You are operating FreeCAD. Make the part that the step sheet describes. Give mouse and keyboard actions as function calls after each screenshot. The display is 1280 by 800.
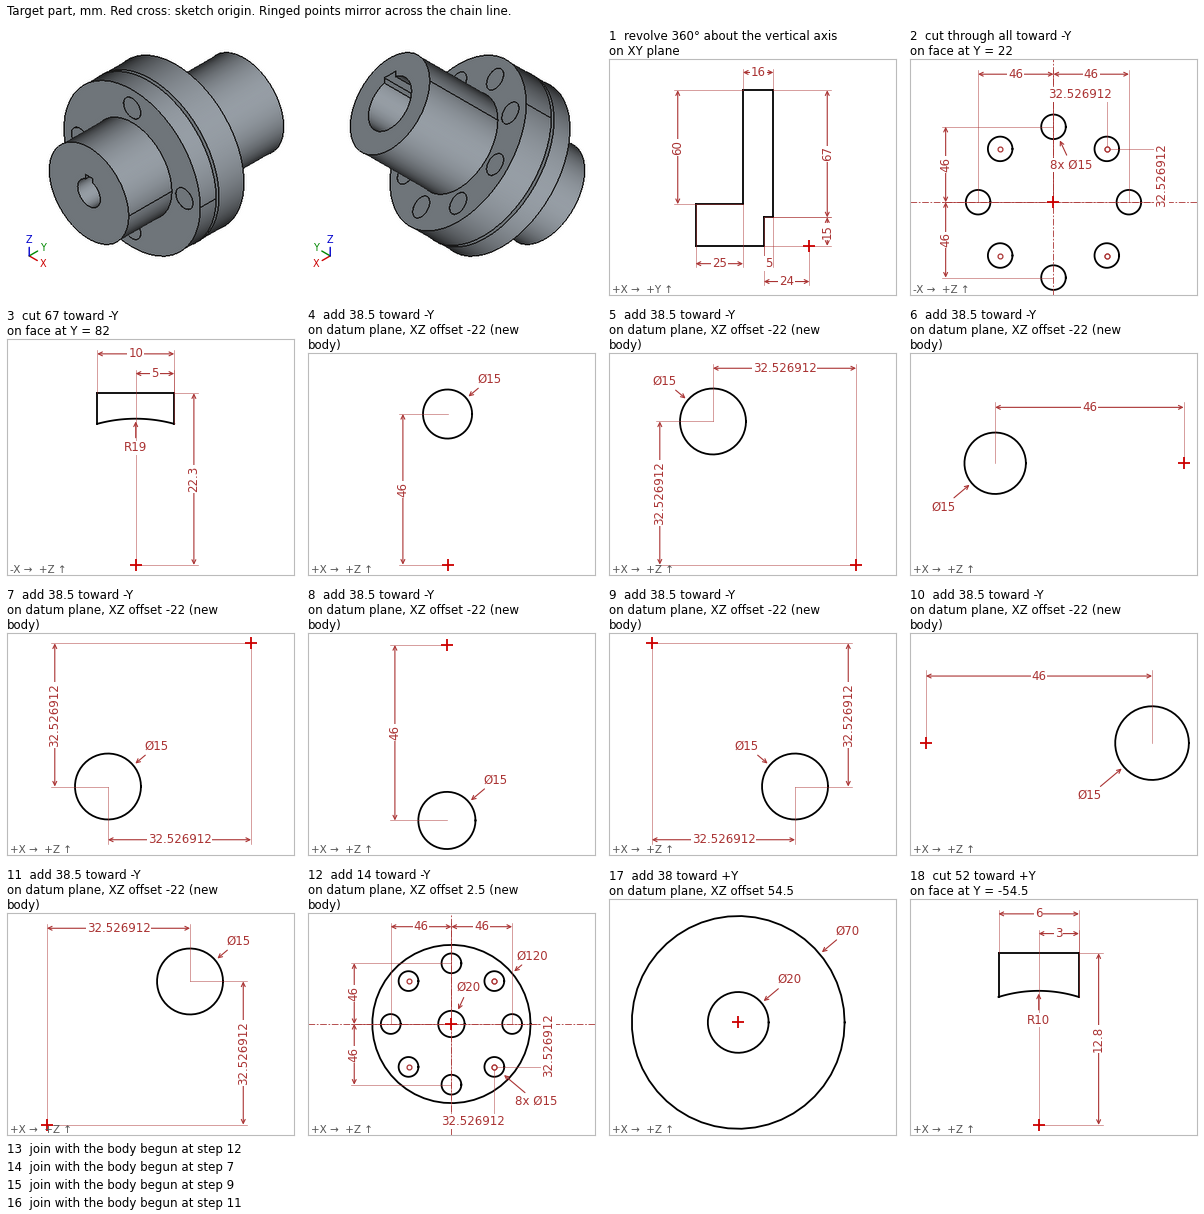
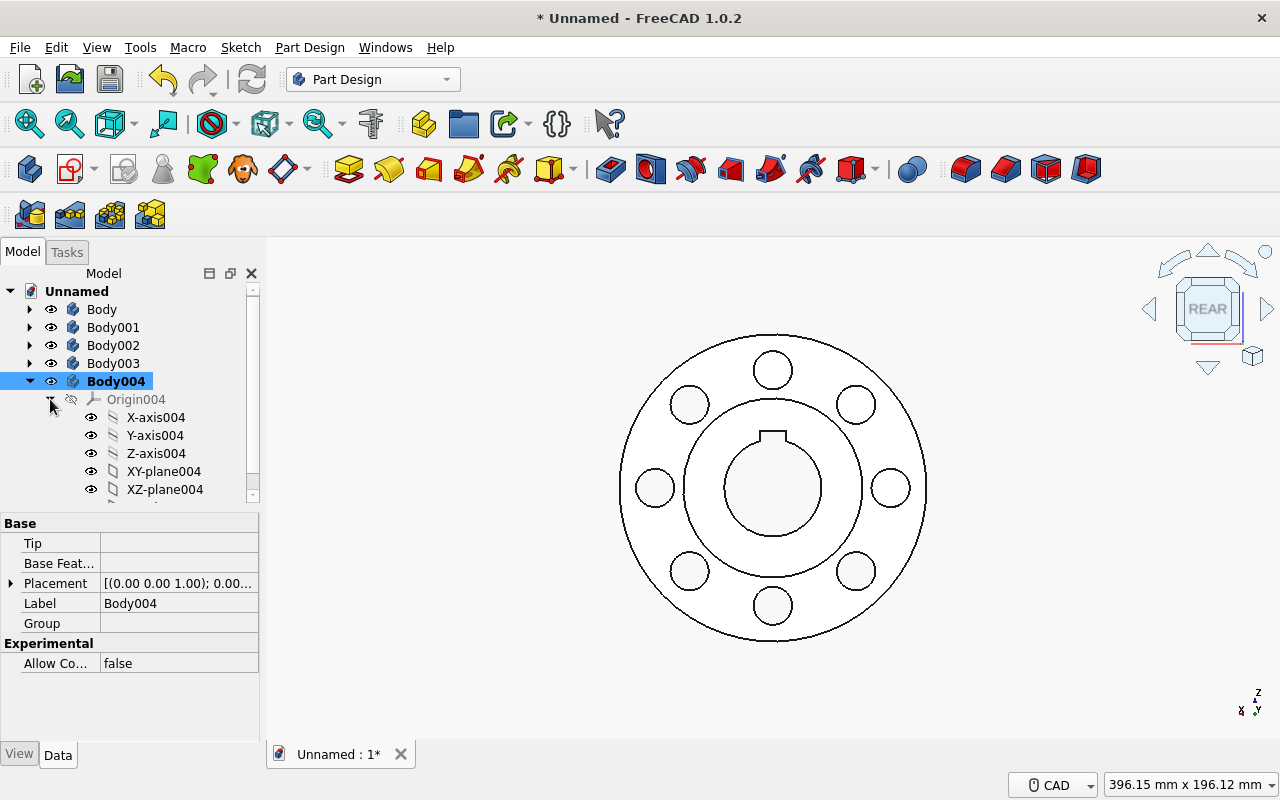
click(136, 489)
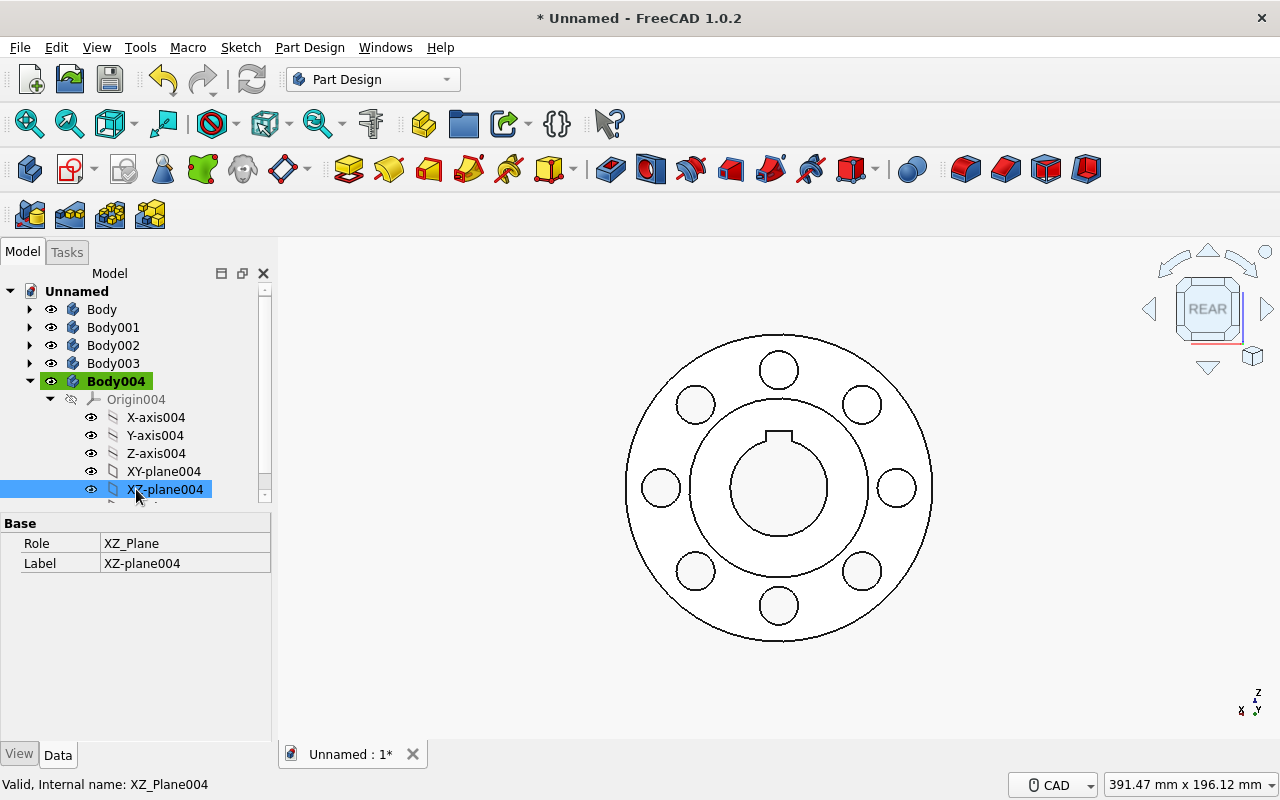
click(284, 170)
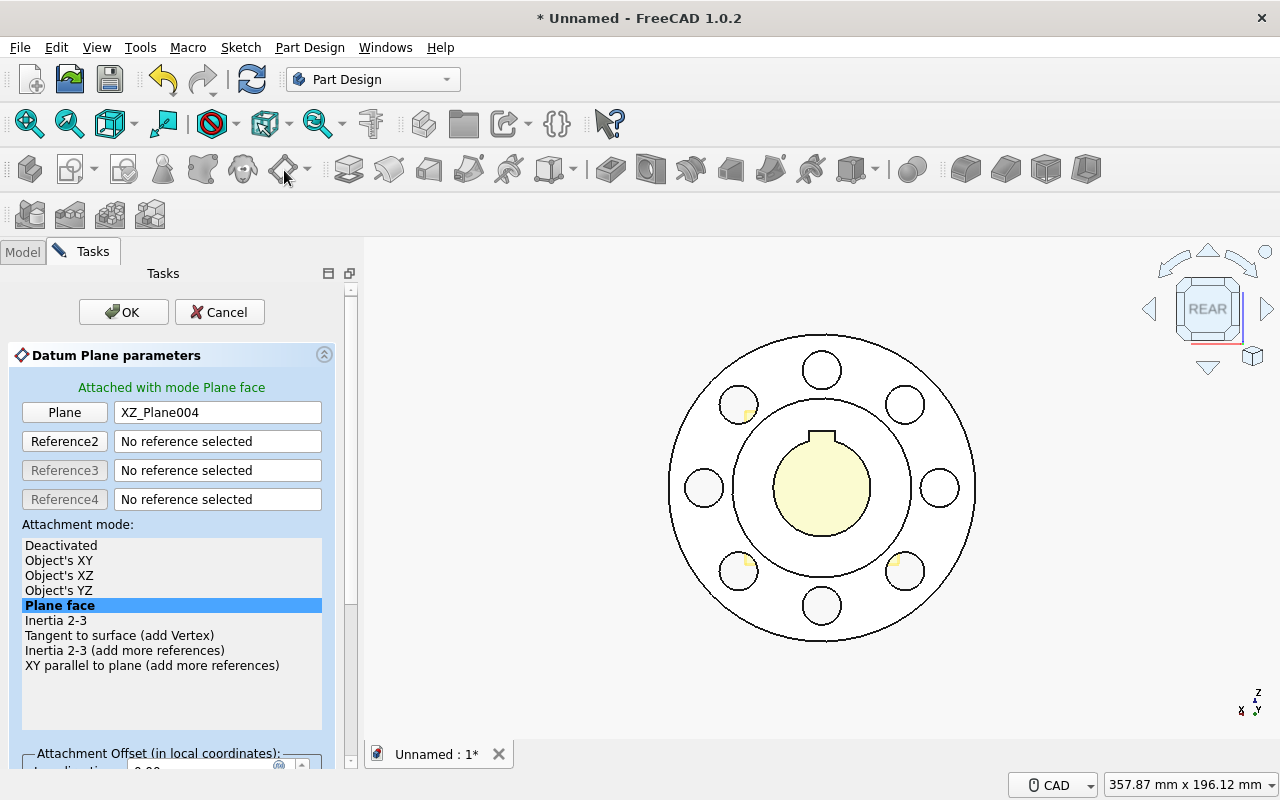
scroll(351, 526, down, 3)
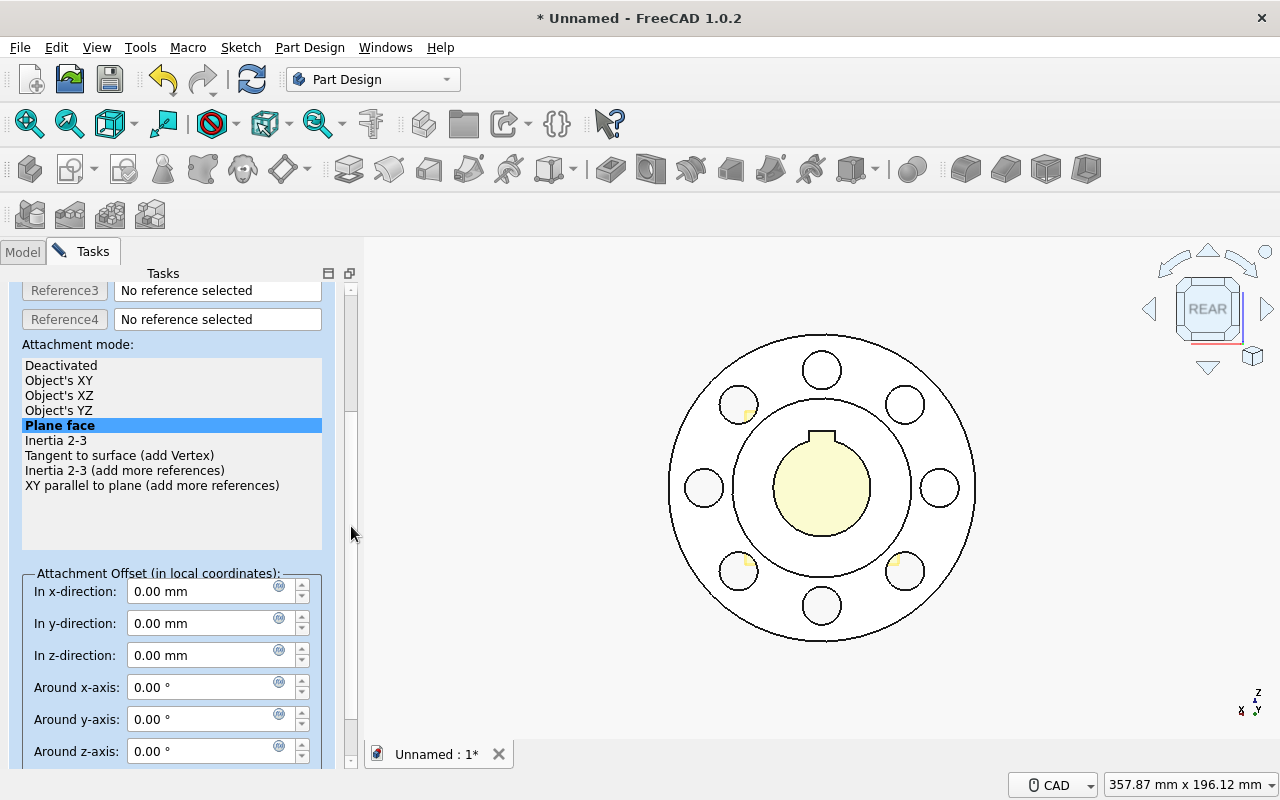
triple_click(210, 655)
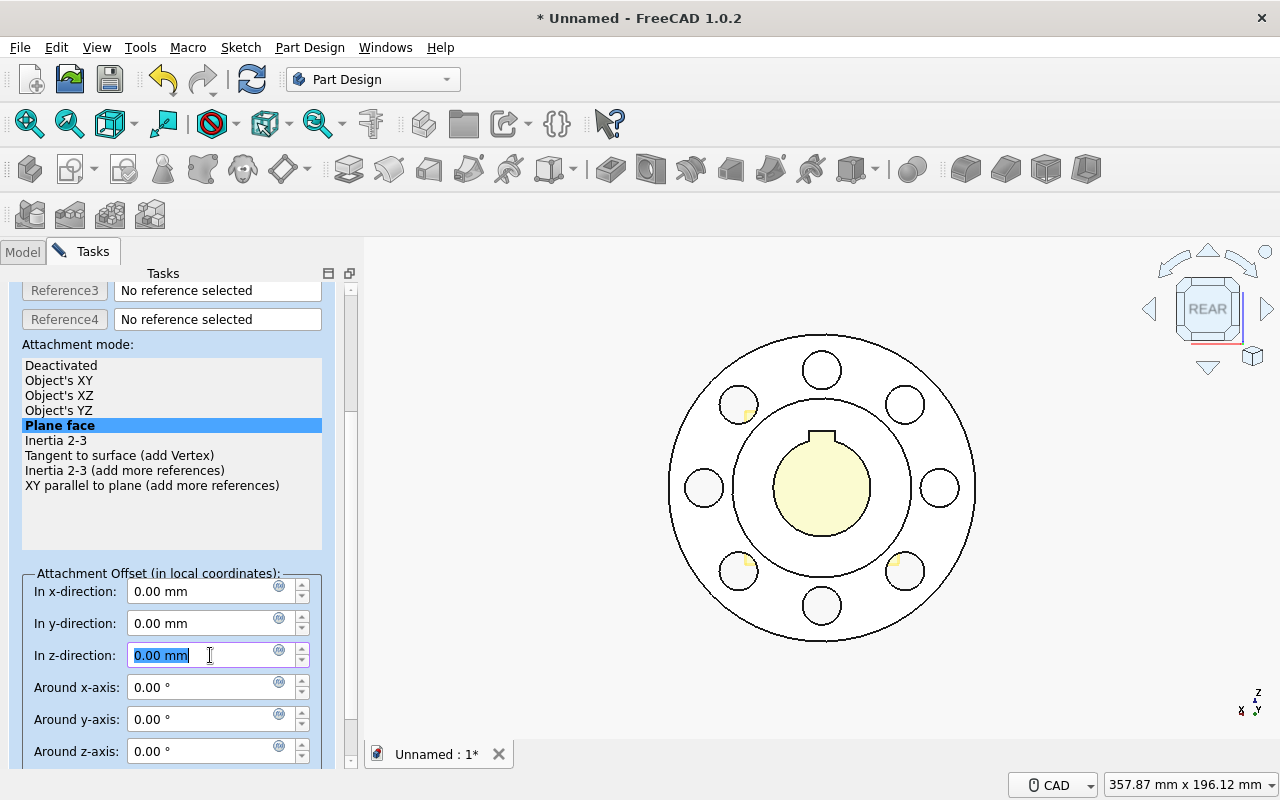
text(-22)
key(Tab)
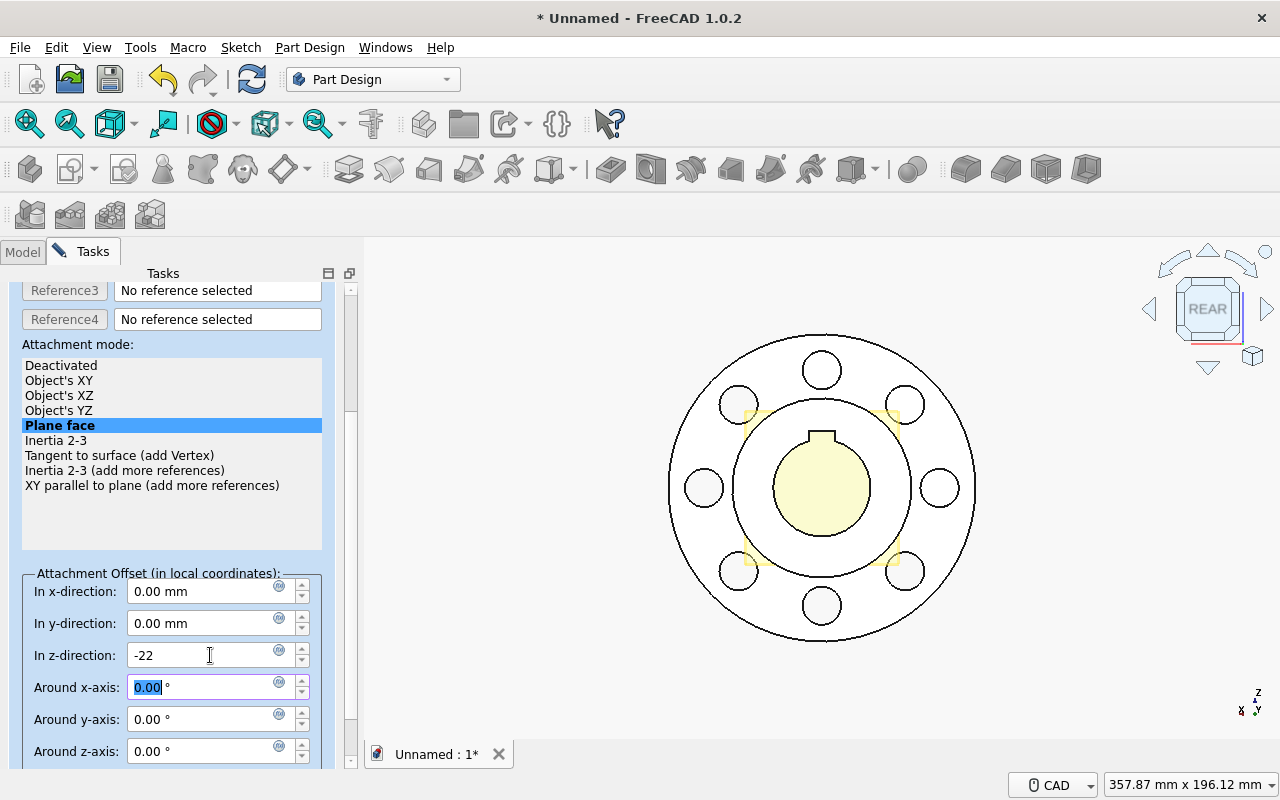
scroll(351, 526, up, 4)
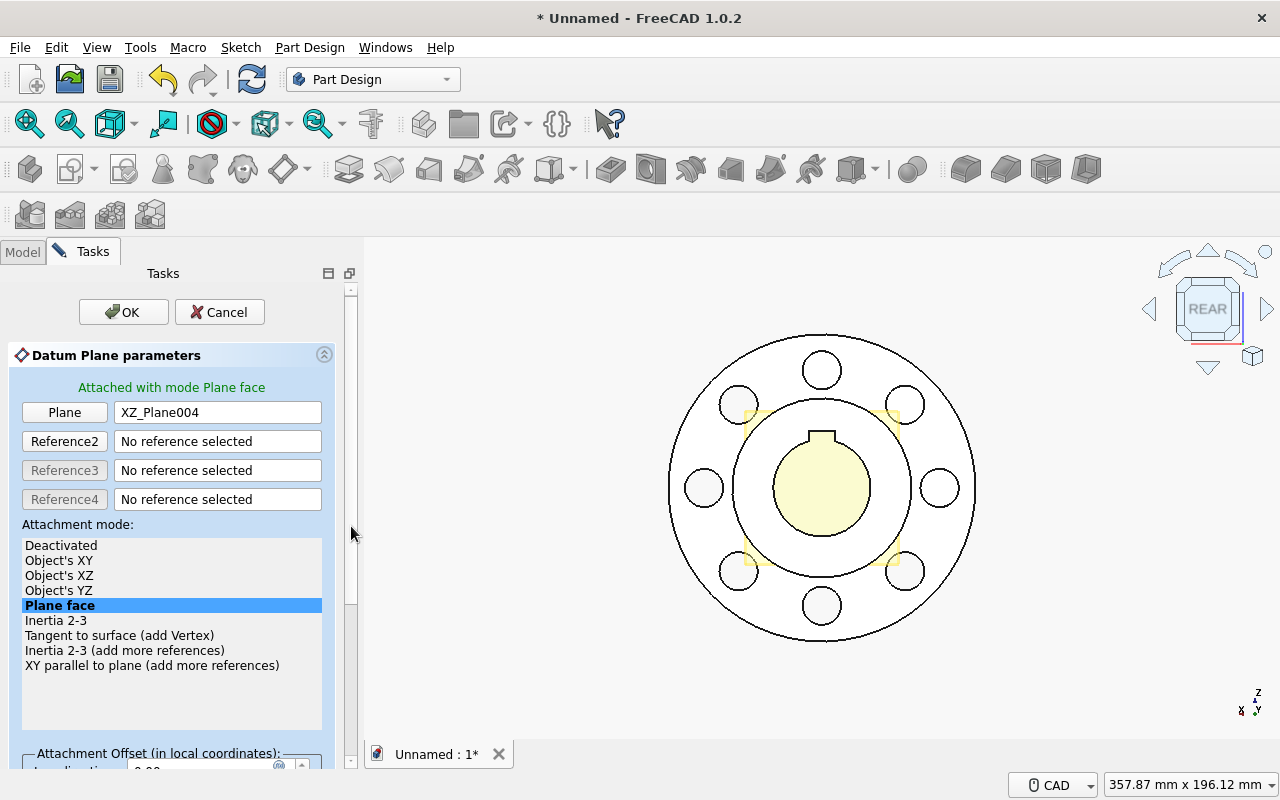
click(124, 312)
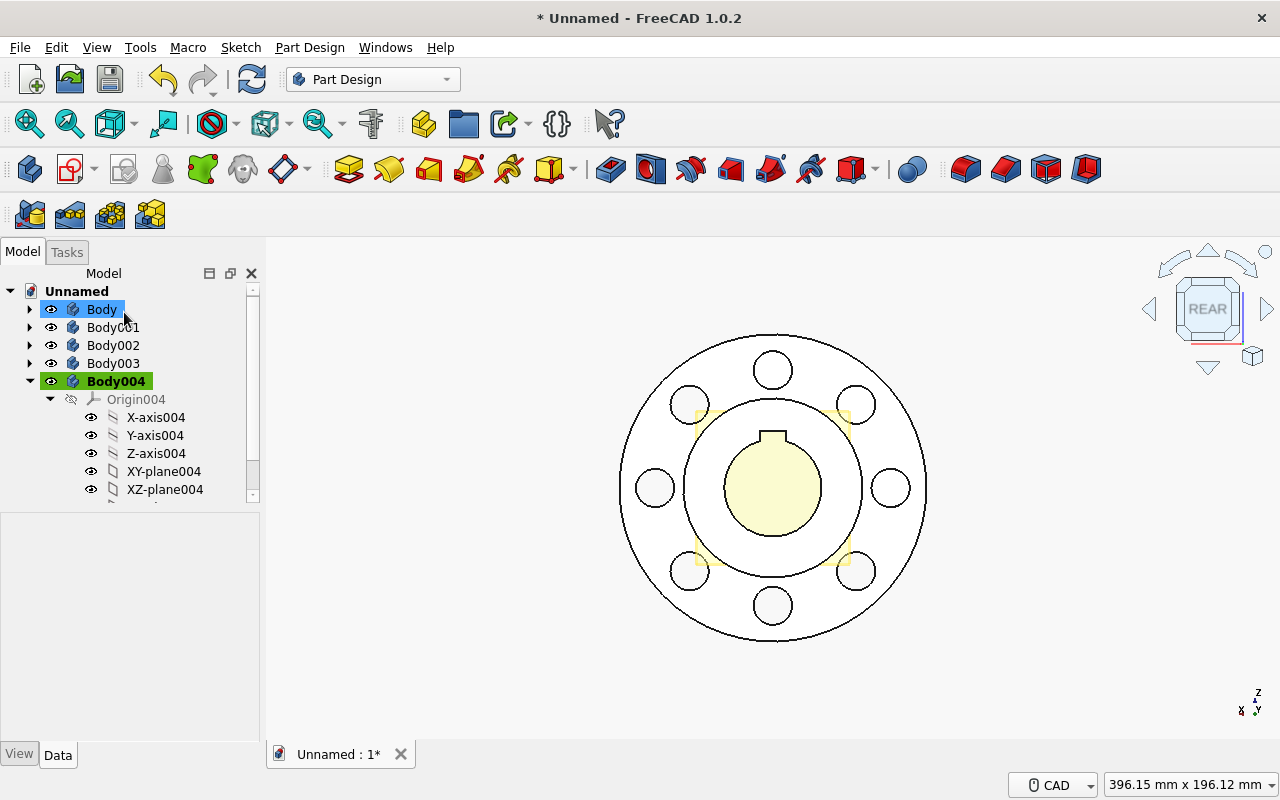
scroll(100, 395, down, 3)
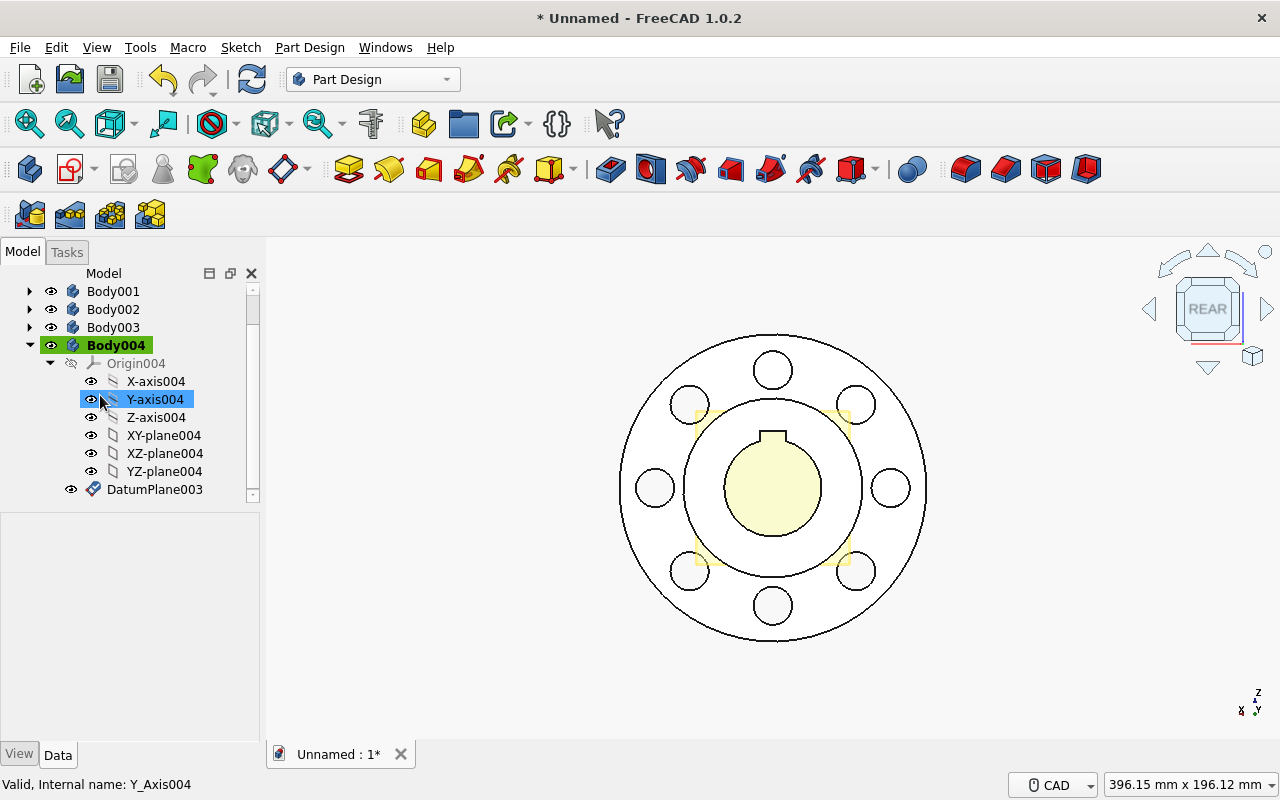
click(116, 489)